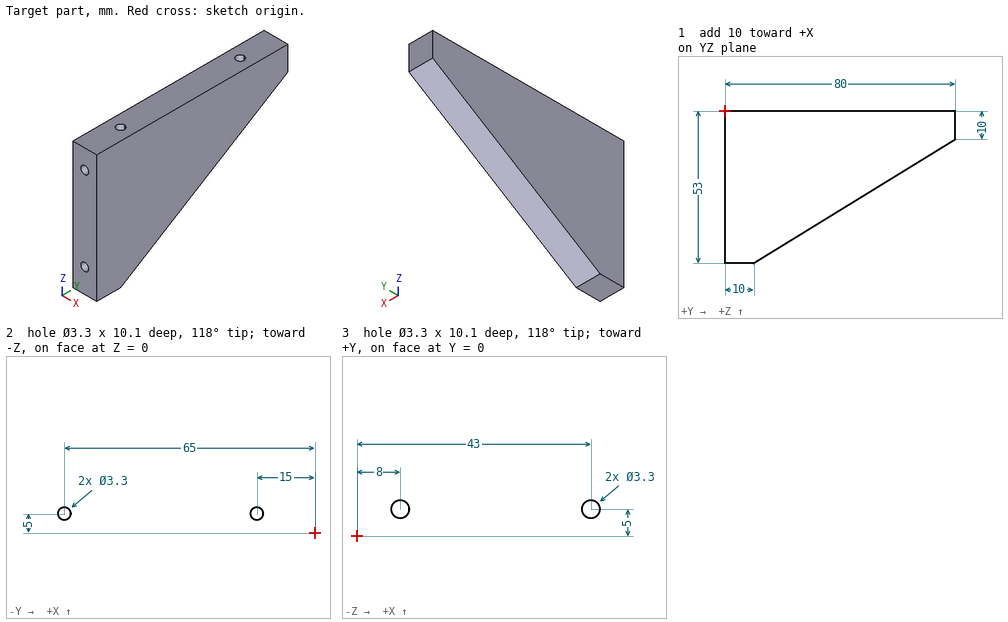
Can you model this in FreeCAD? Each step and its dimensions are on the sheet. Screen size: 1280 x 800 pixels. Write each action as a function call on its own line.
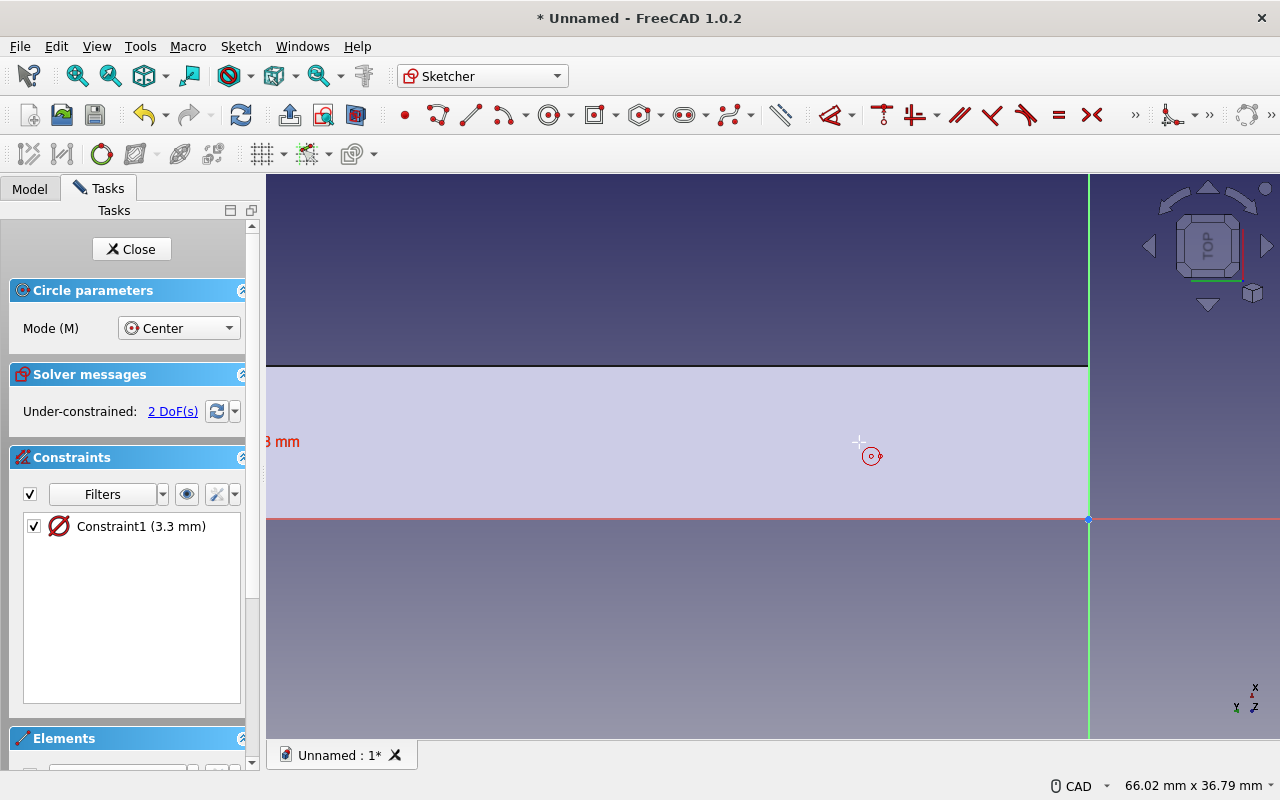
click(859, 442)
move(876, 424)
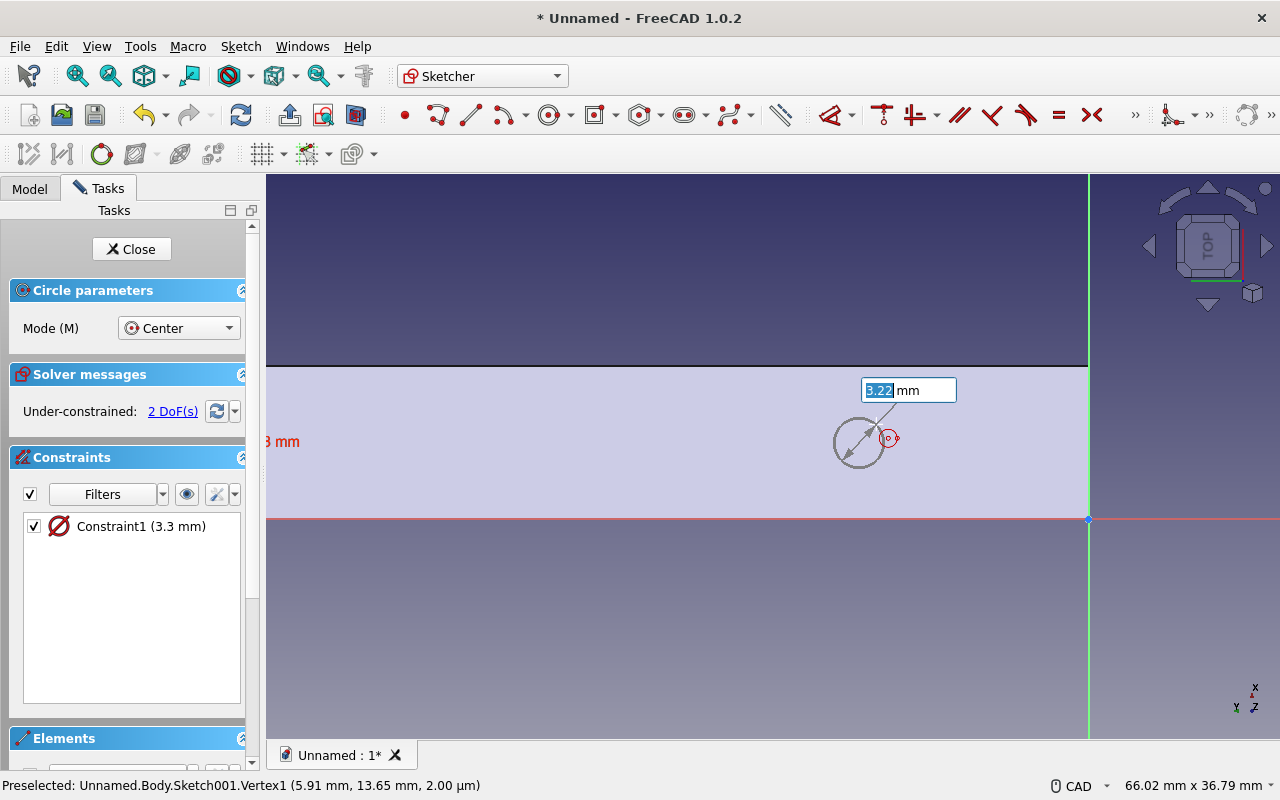
text(3.3)
key(Return)
key(Escape)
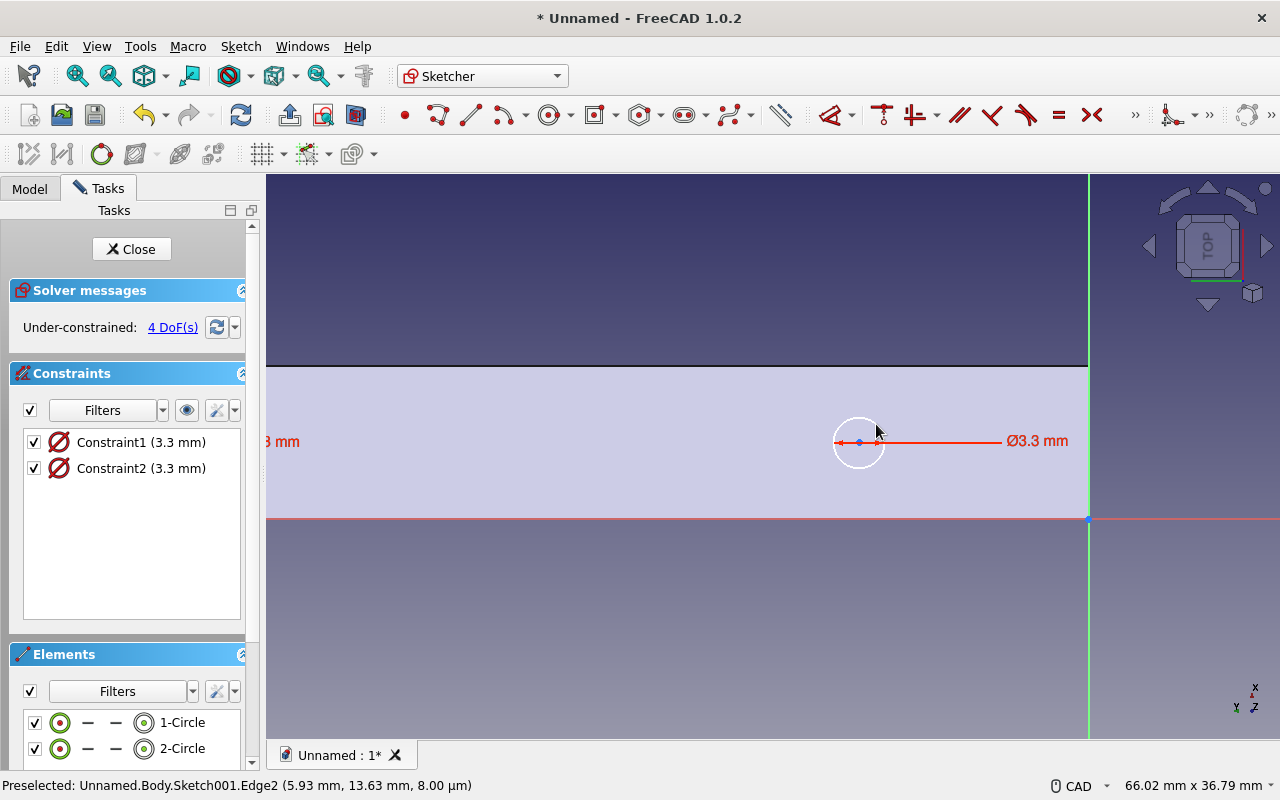
scroll(859, 442, down, 3)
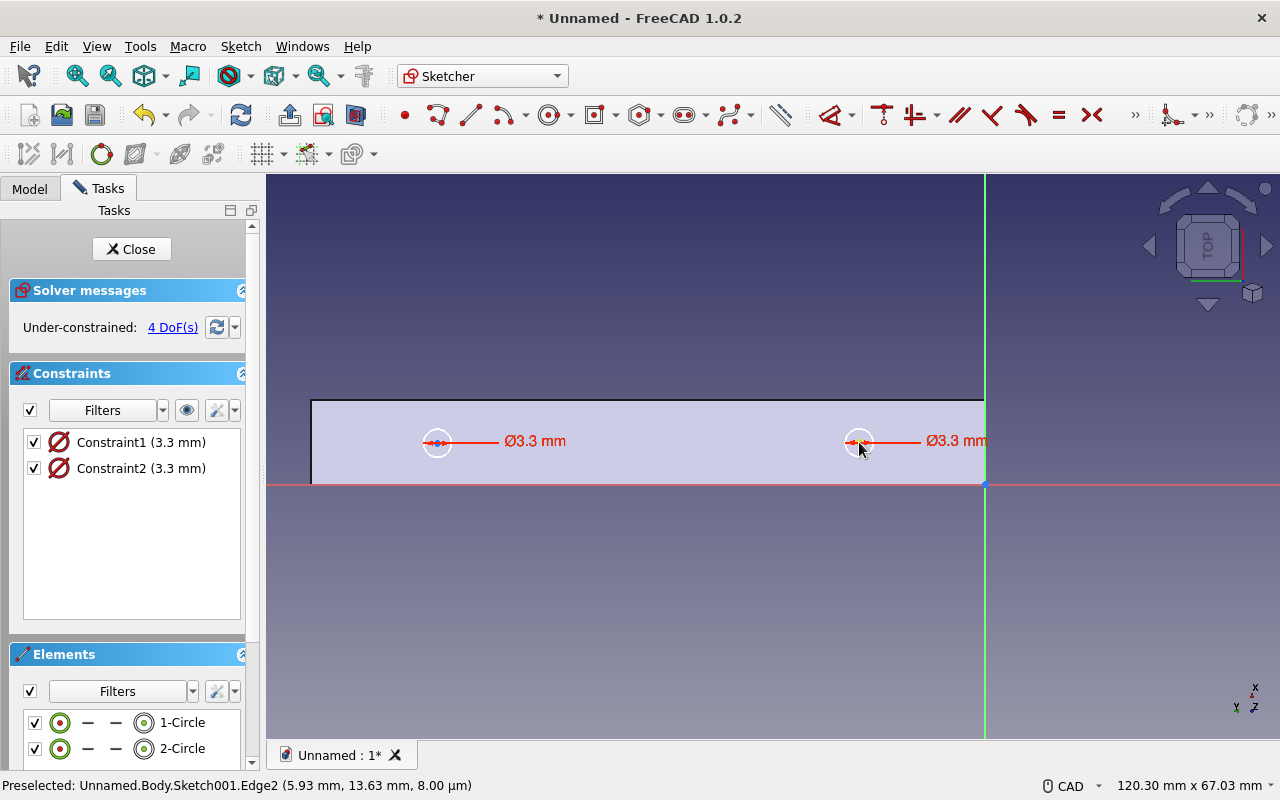
click(438, 443)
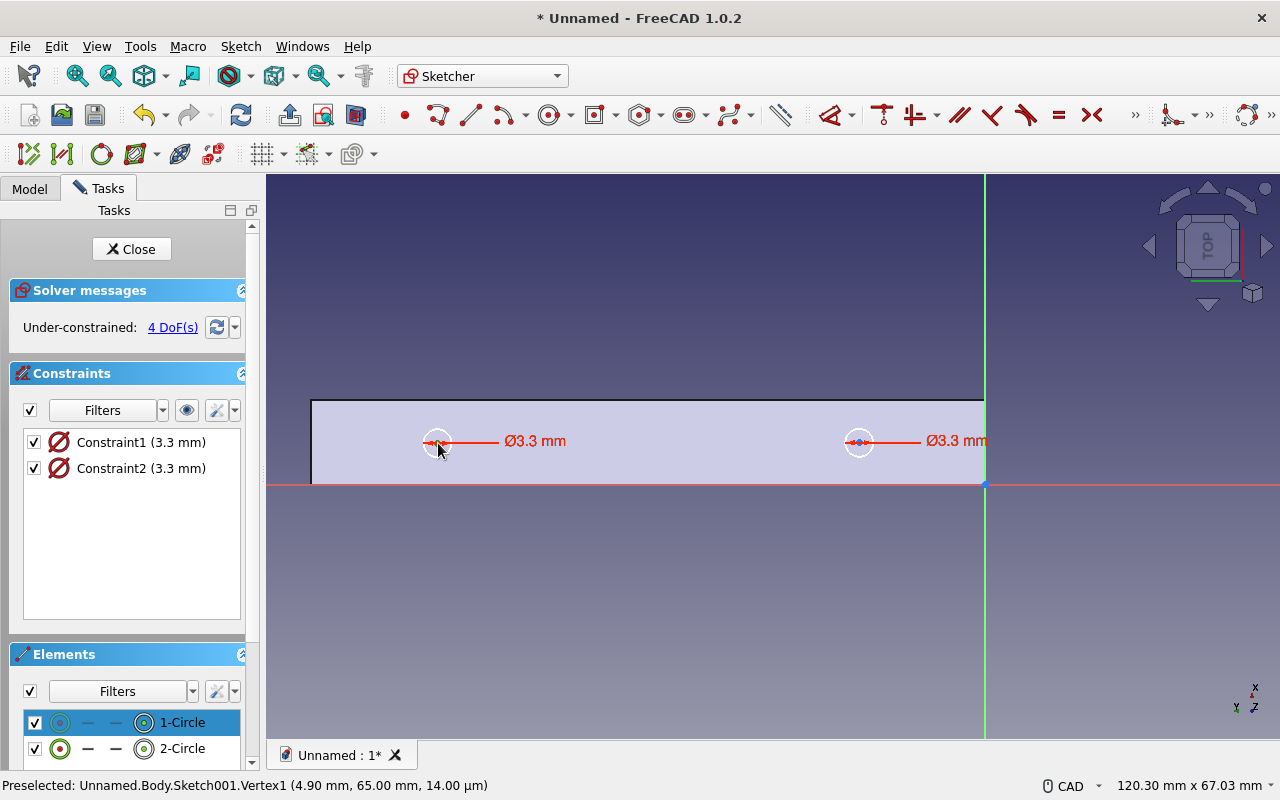
click(859, 443)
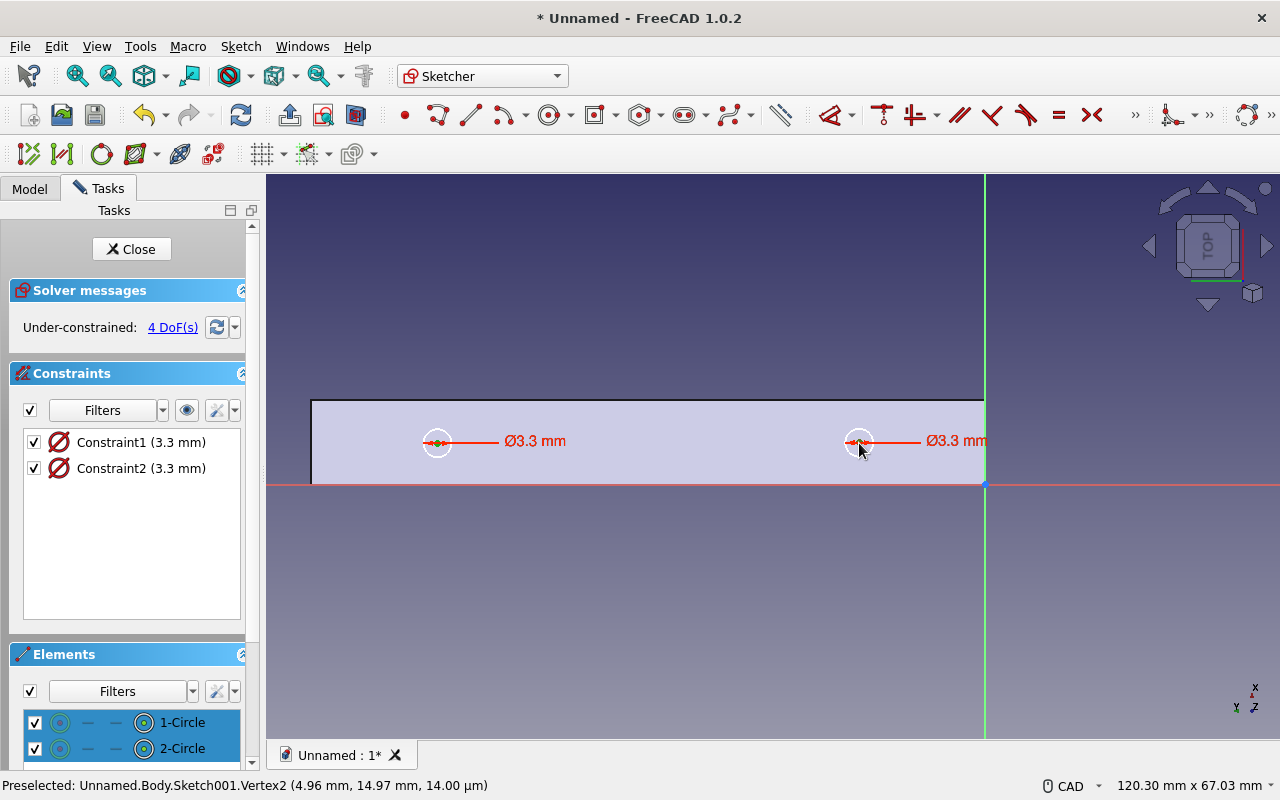
key(h)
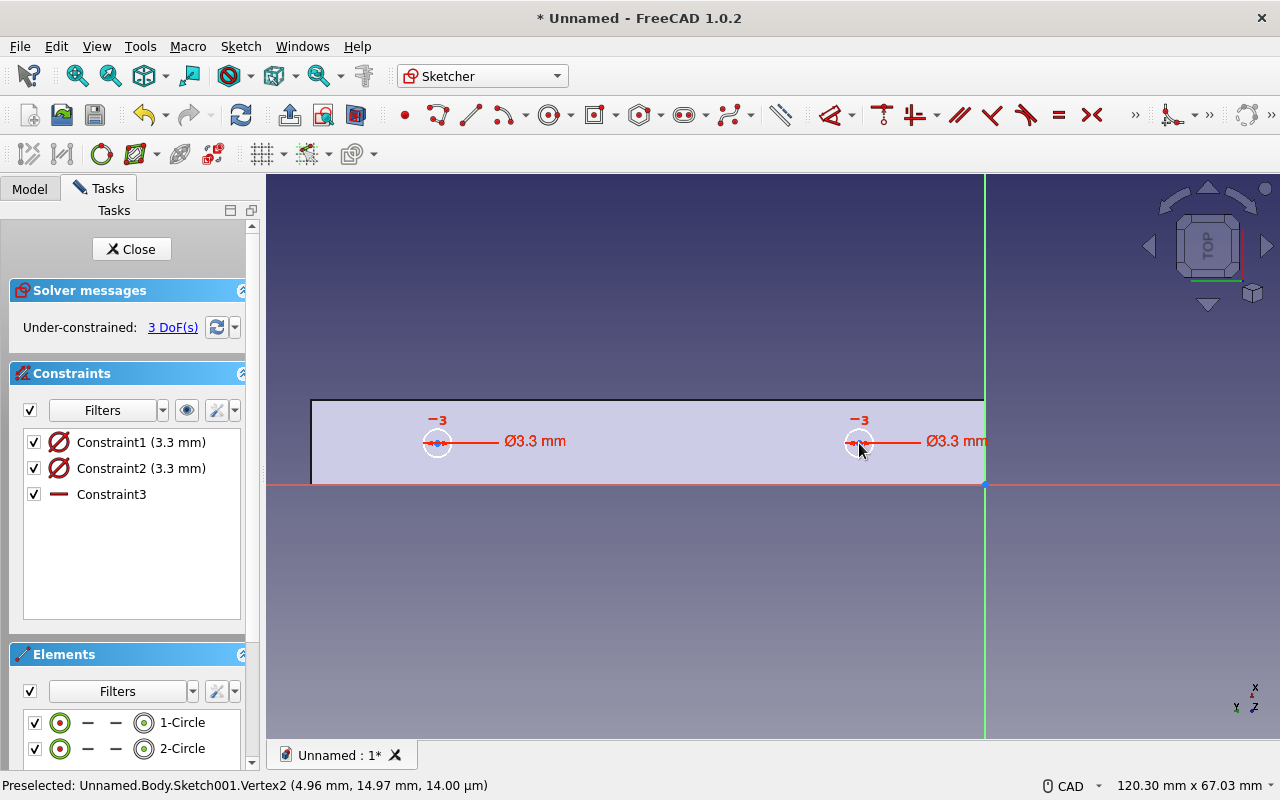
click(830, 116)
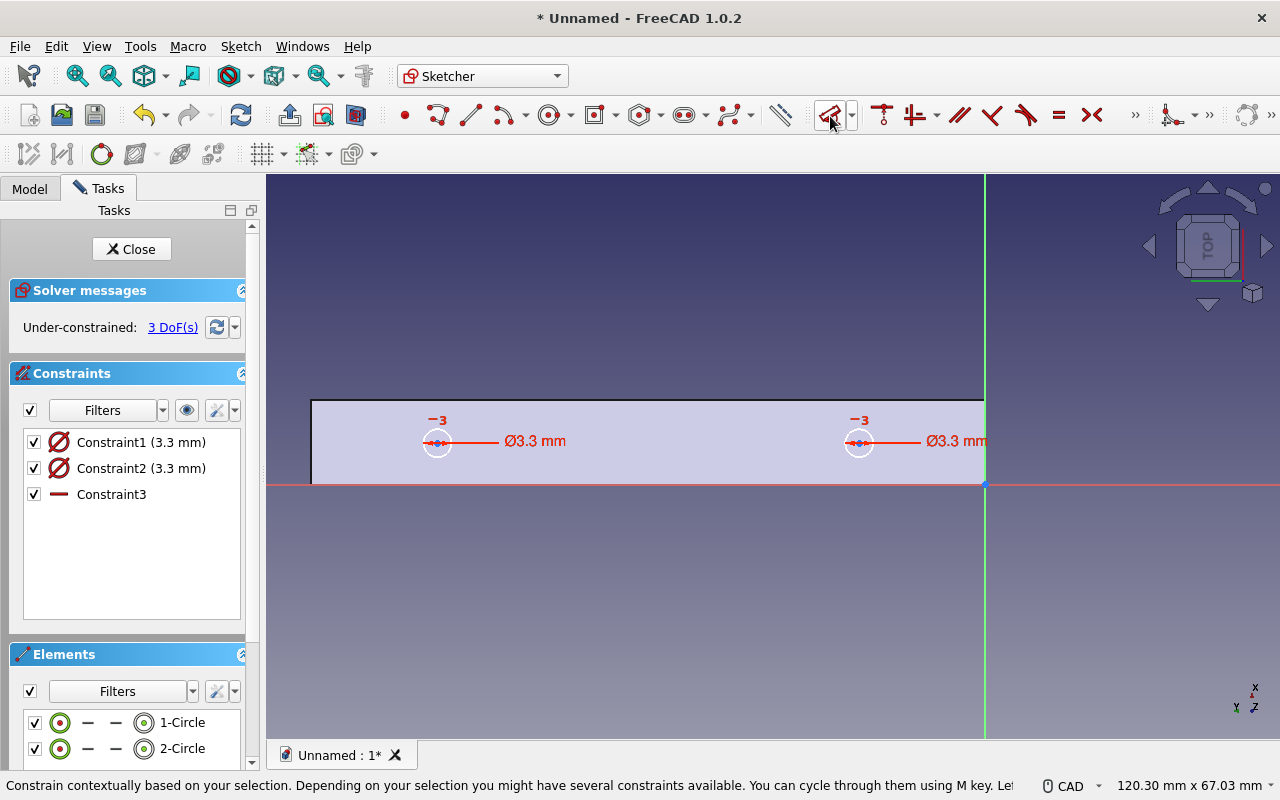
click(438, 443)
click(1019, 464)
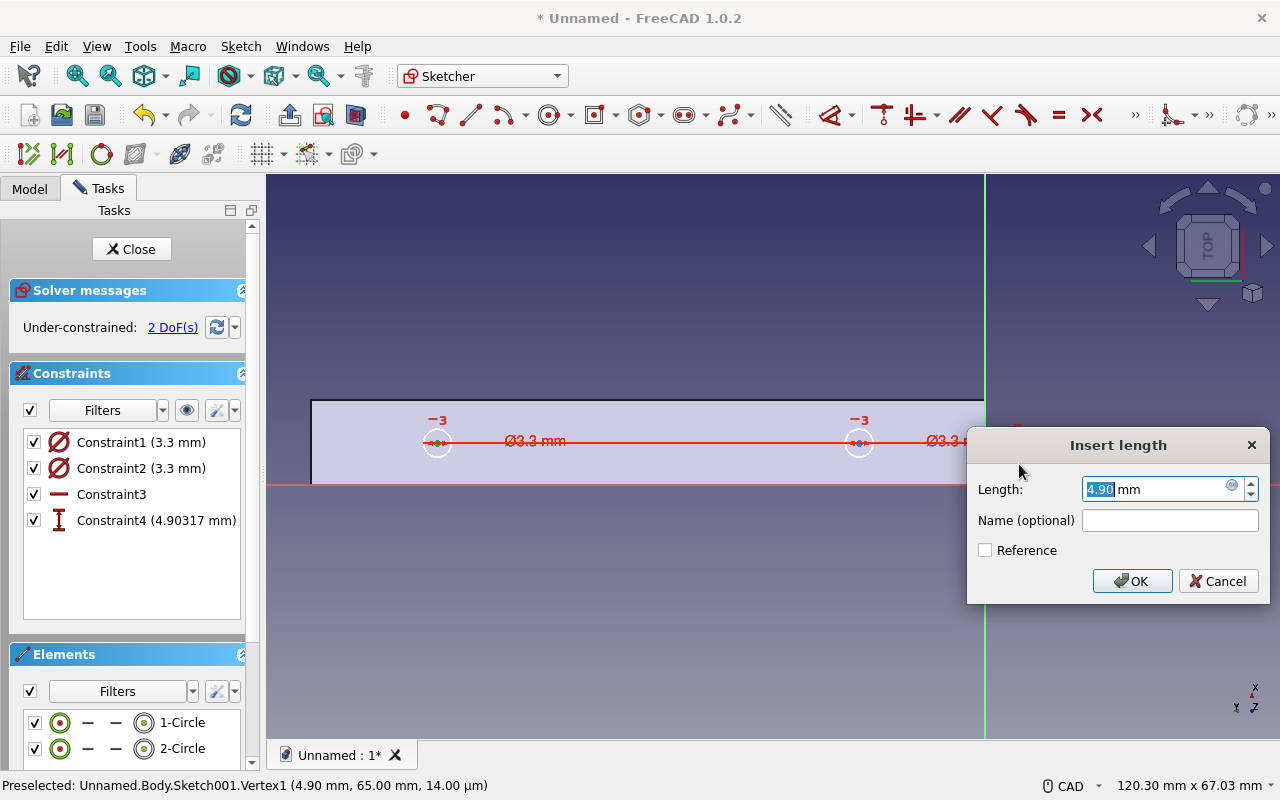
text(5)
key(Return)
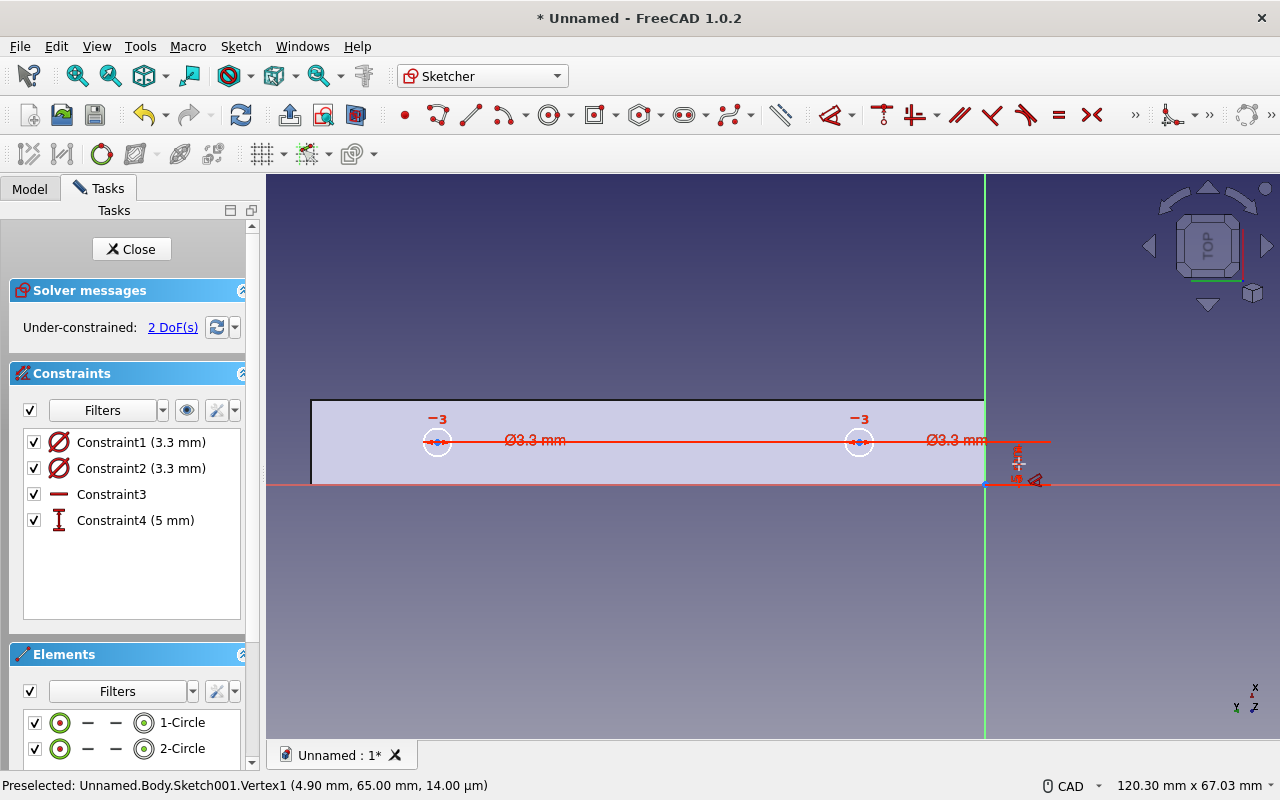
click(438, 442)
click(711, 519)